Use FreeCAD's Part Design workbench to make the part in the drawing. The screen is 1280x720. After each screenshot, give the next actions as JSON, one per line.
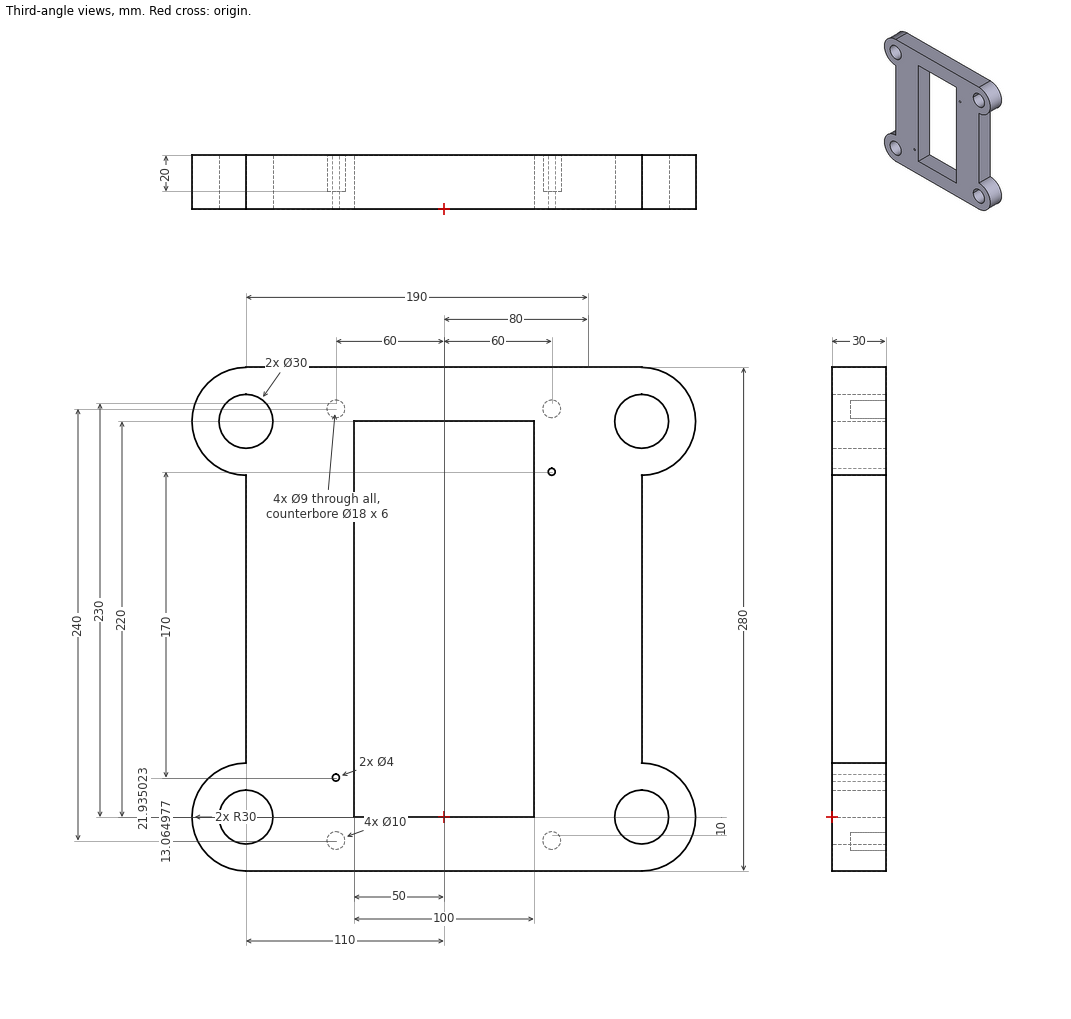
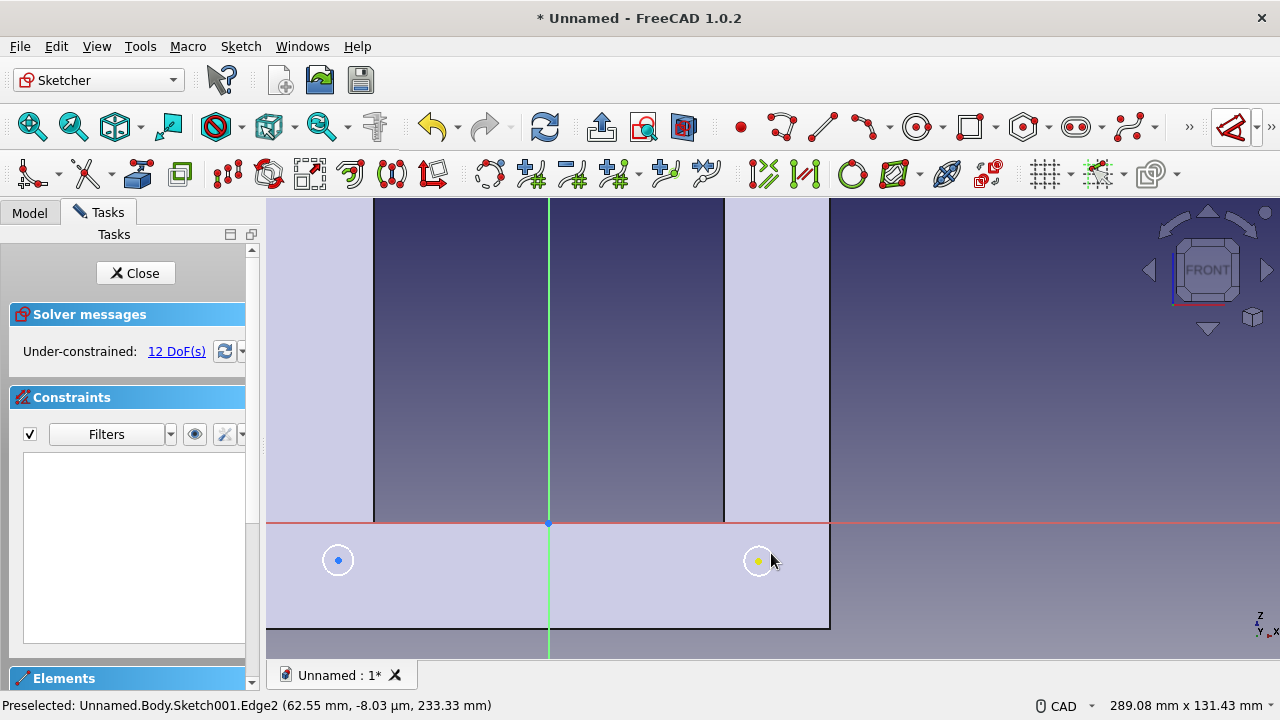
{"action": "left_click", "coordinate": [769, 551]}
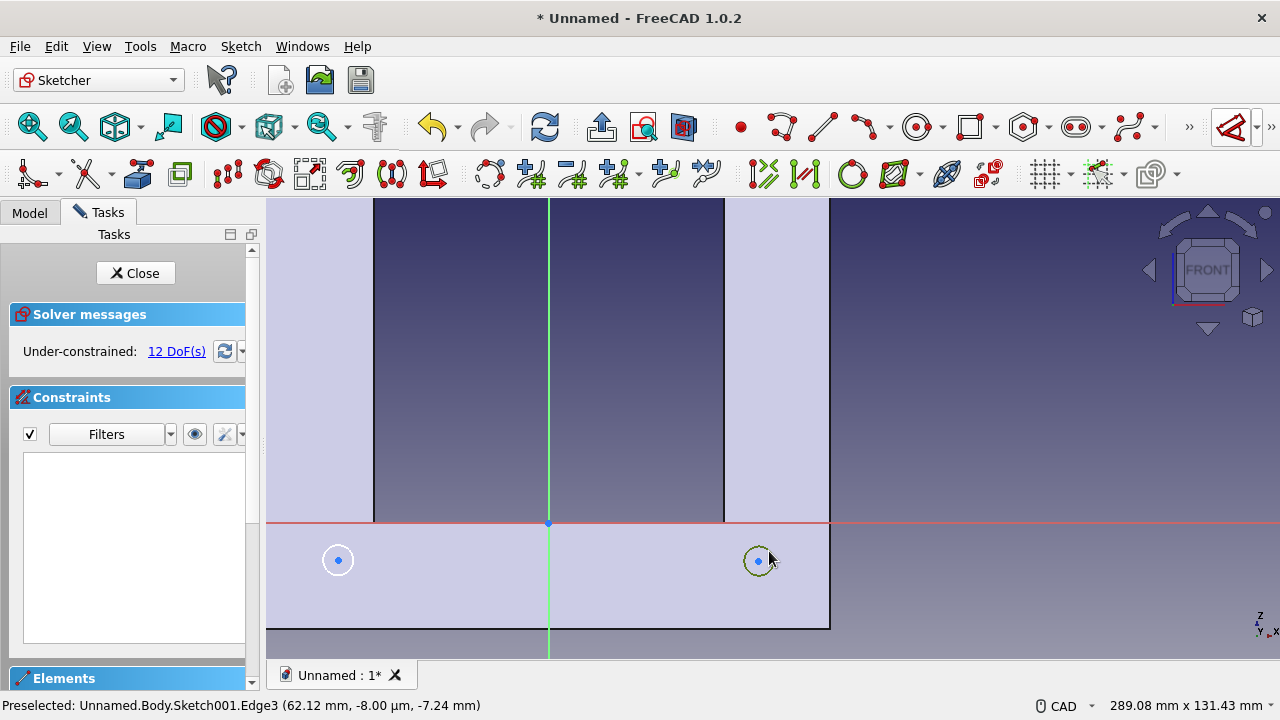
{"action": "left_click", "coordinate": [349, 550]}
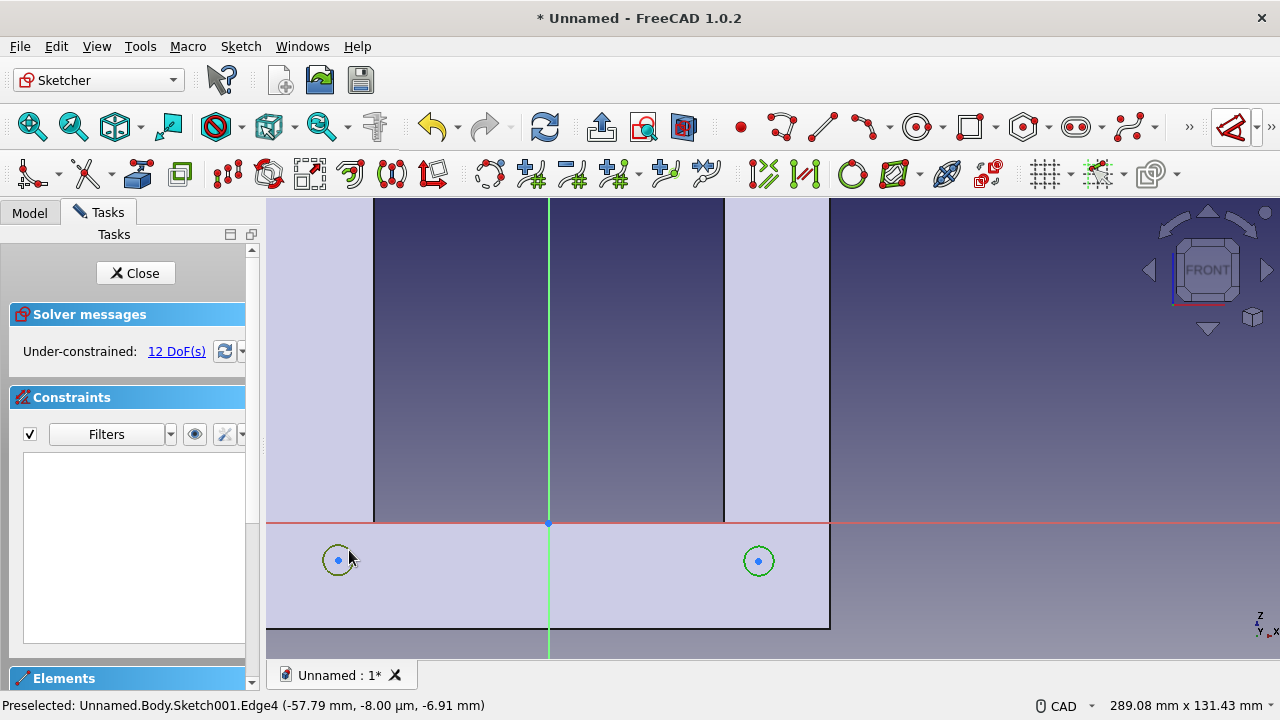
{"action": "key", "text": "e"}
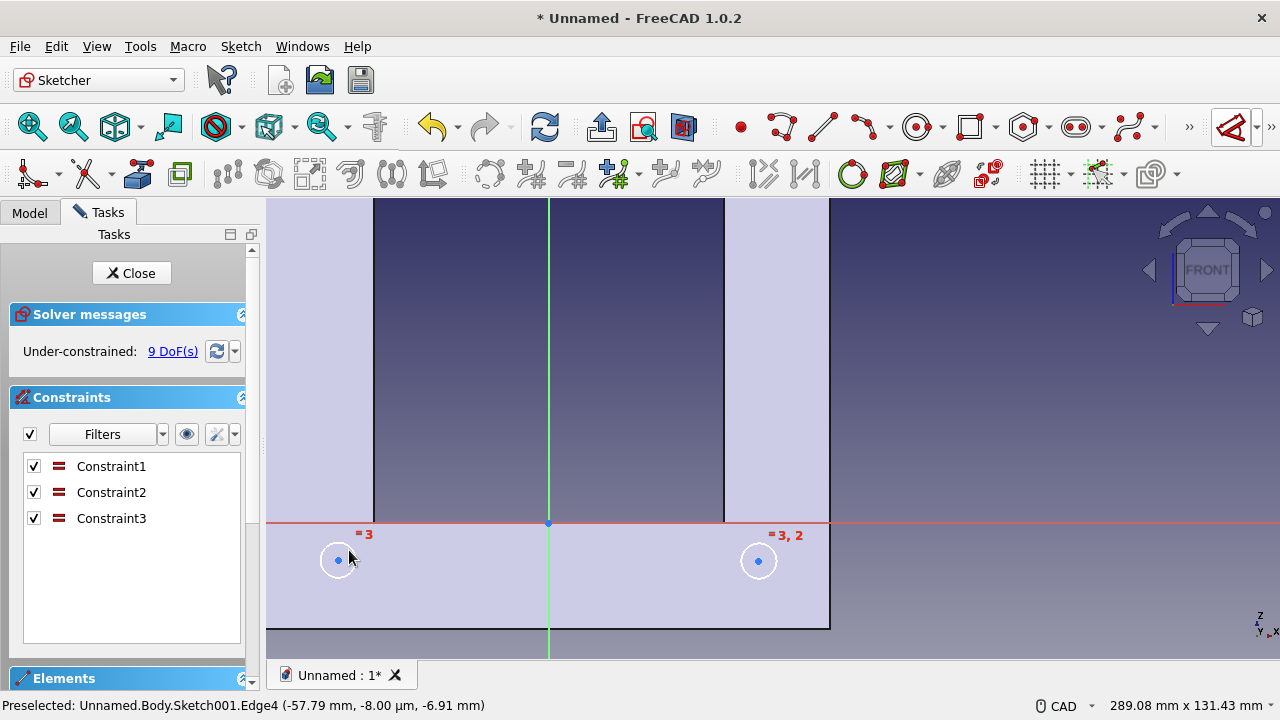
{"action": "left_click", "coordinate": [1230, 128]}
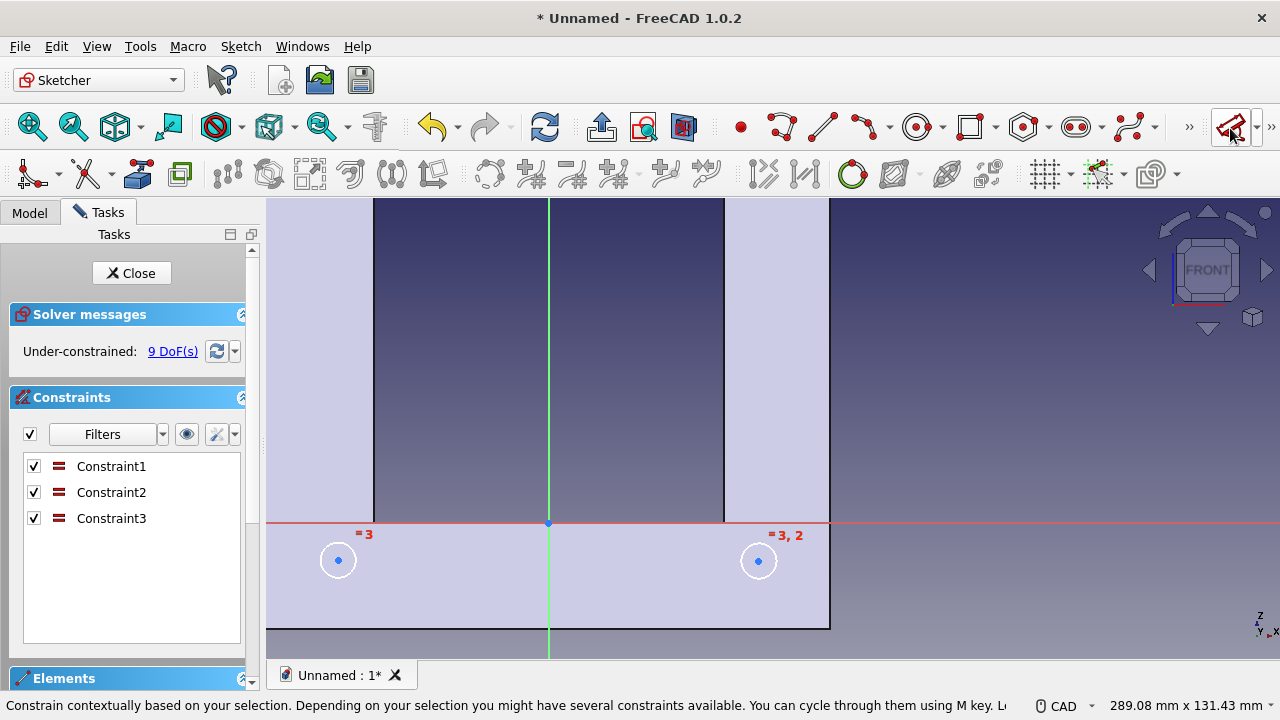
{"action": "scroll", "coordinate": [772, 554], "scroll_direction": "down", "scroll_amount": 6}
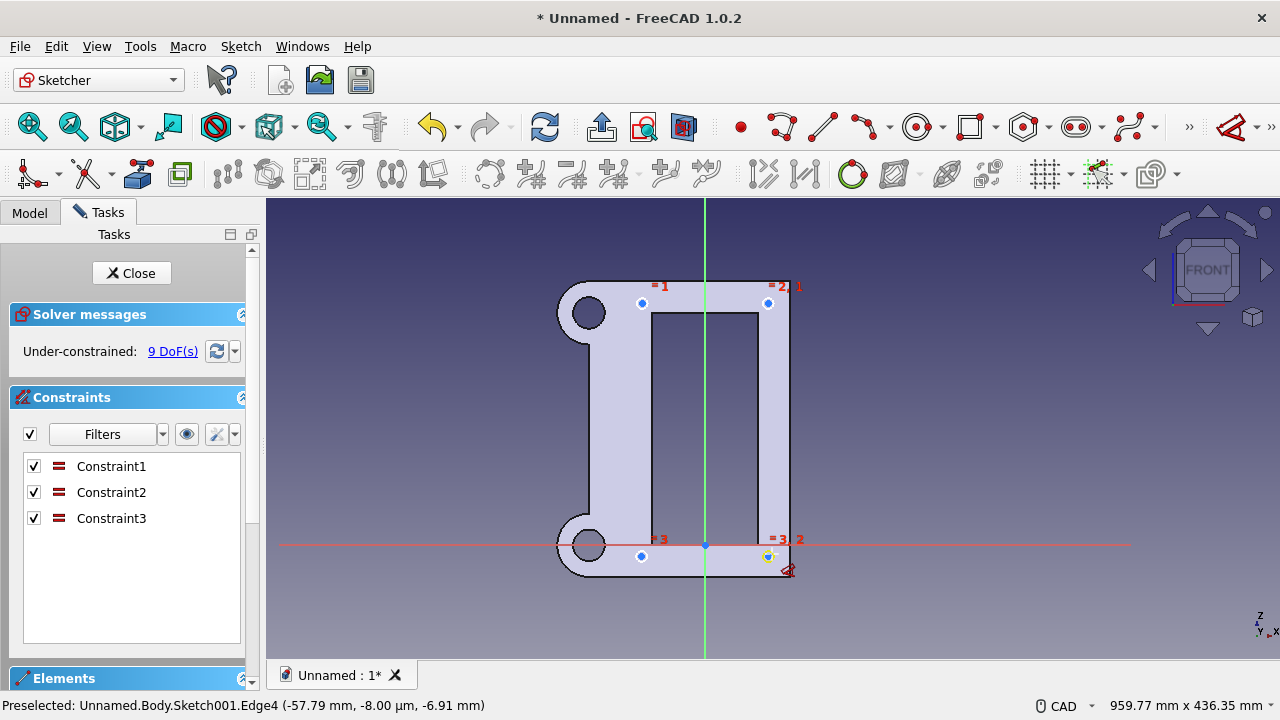
{"action": "scroll", "coordinate": [646, 300], "scroll_direction": "up", "scroll_amount": 8}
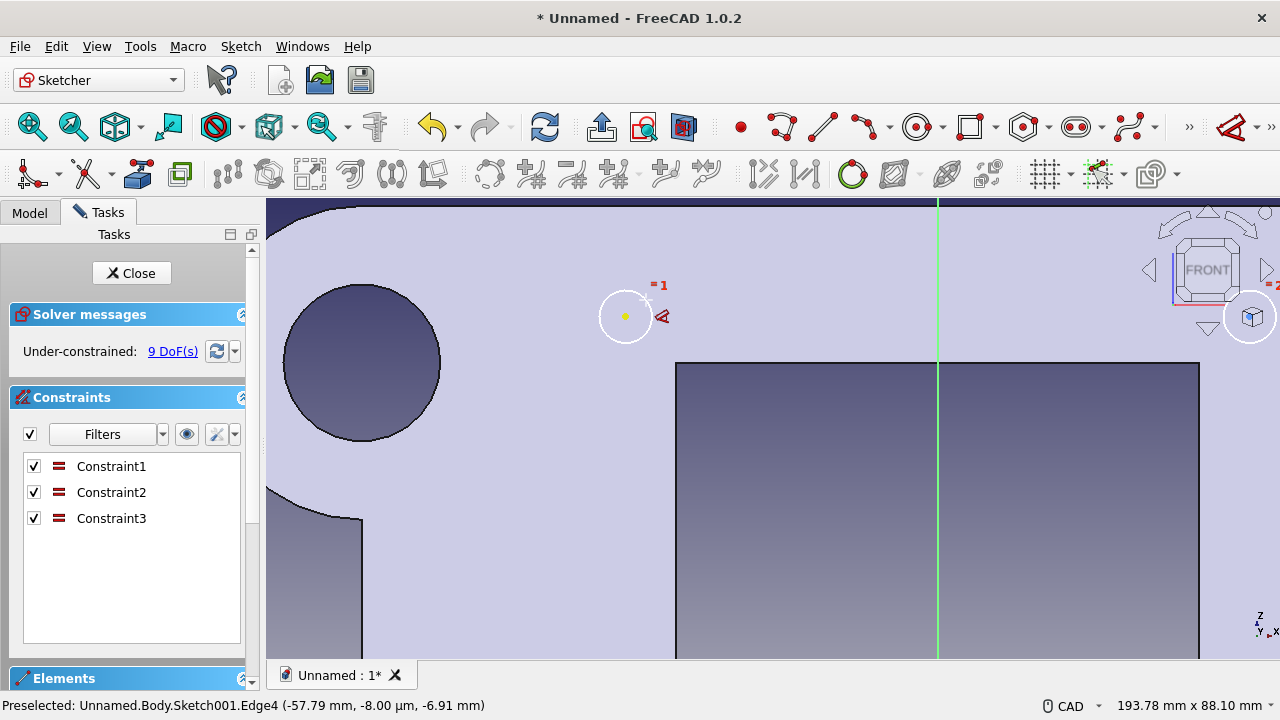
{"action": "left_click", "coordinate": [644, 298]}
{"action": "left_click", "coordinate": [666, 275]}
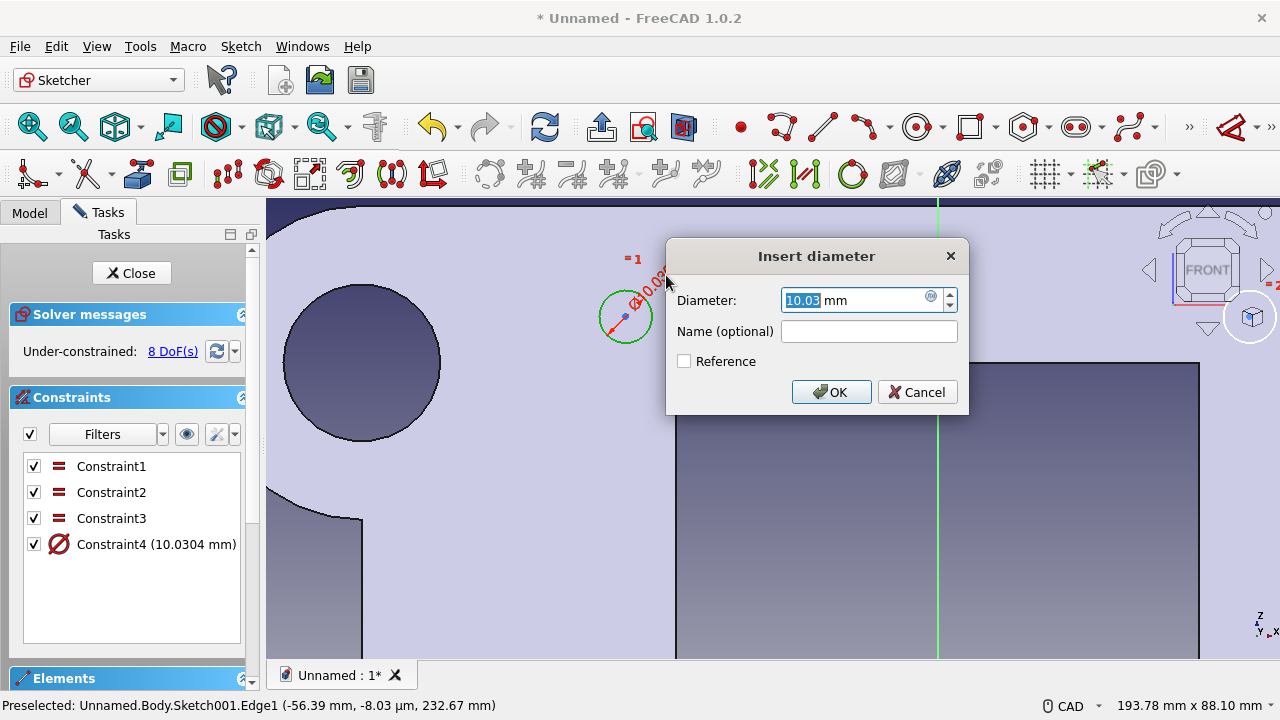
{"action": "type", "text": "9"}
{"action": "key", "text": "Return"}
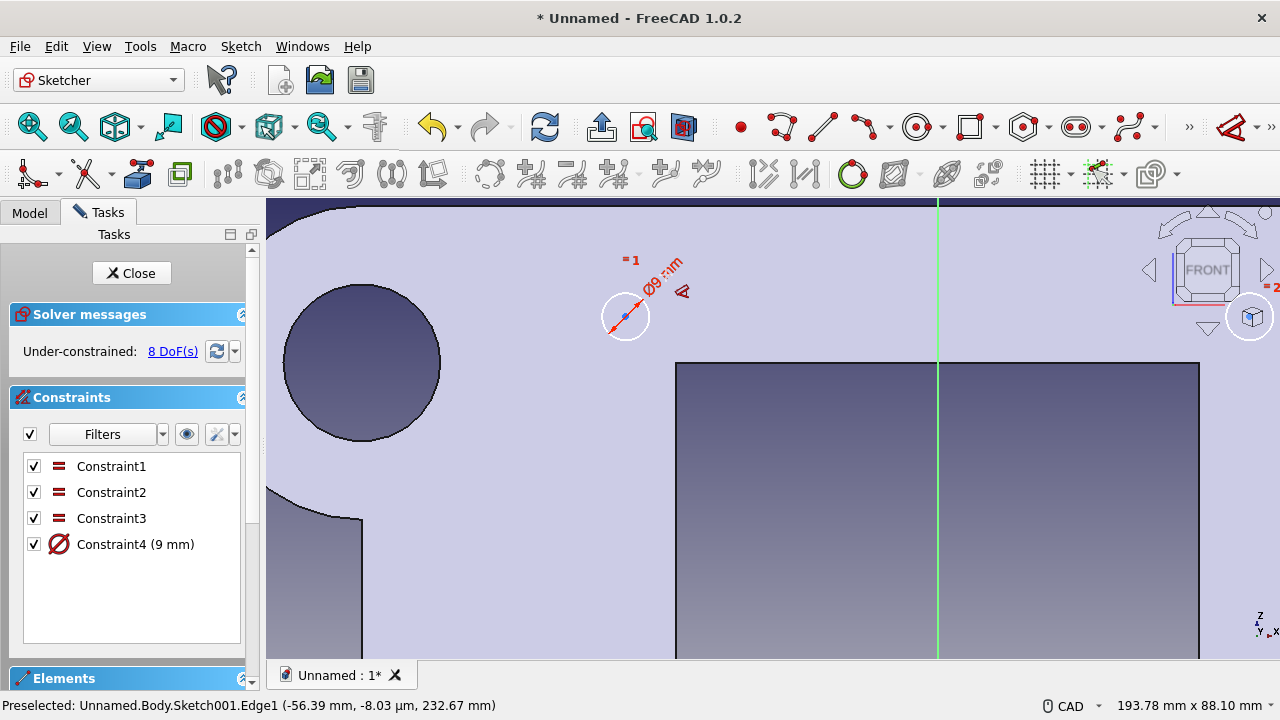
{"action": "scroll", "coordinate": [646, 300], "scroll_direction": "down", "scroll_amount": 8}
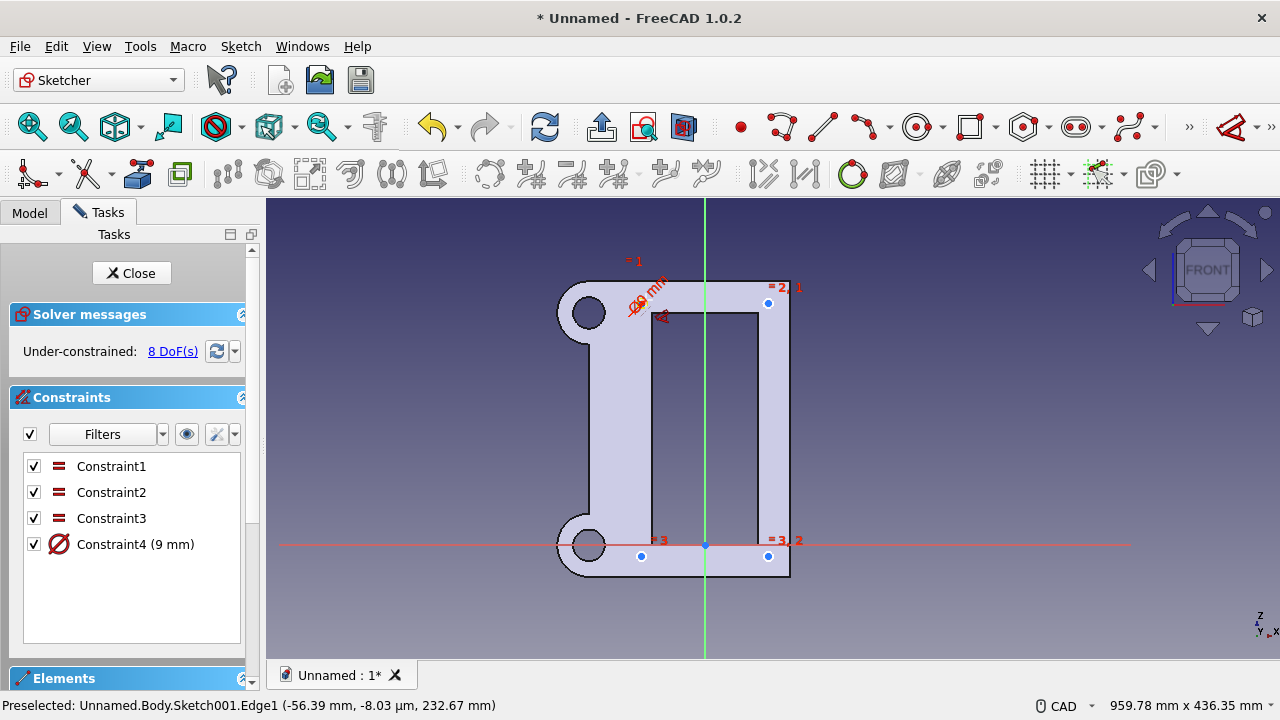
{"action": "left_click", "coordinate": [642, 304]}
{"action": "left_click", "coordinate": [674, 270]}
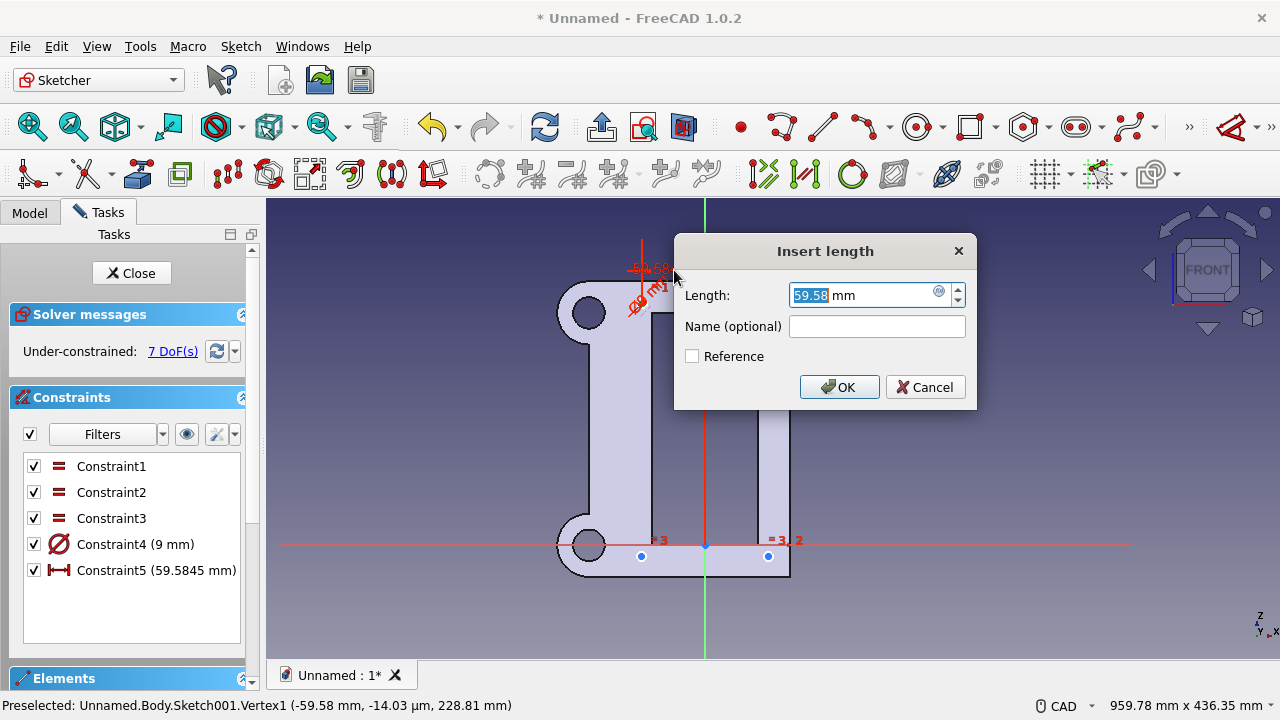
{"action": "type", "text": "60"}
{"action": "key", "text": "Return"}